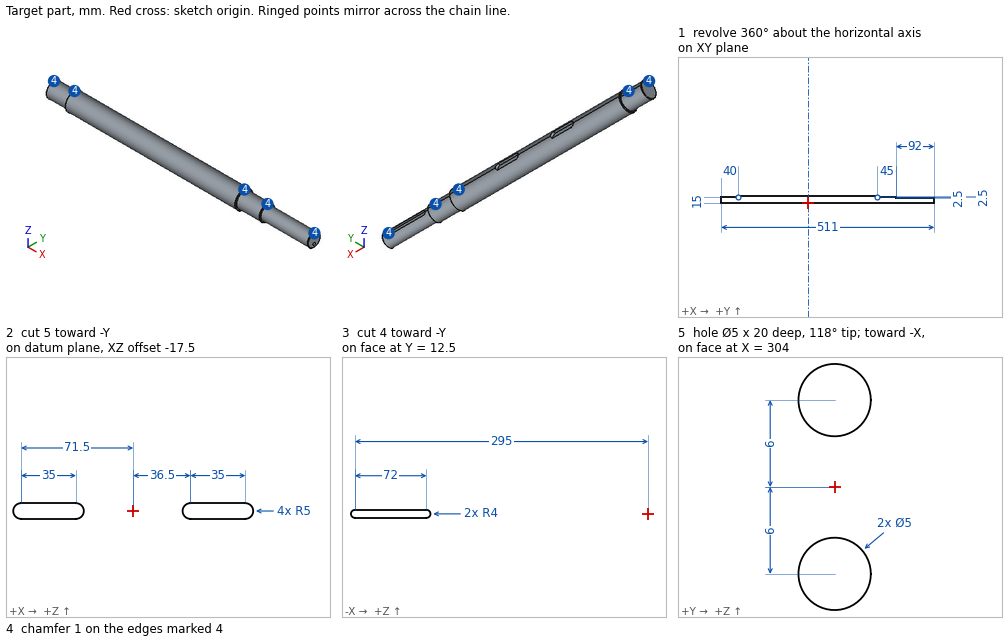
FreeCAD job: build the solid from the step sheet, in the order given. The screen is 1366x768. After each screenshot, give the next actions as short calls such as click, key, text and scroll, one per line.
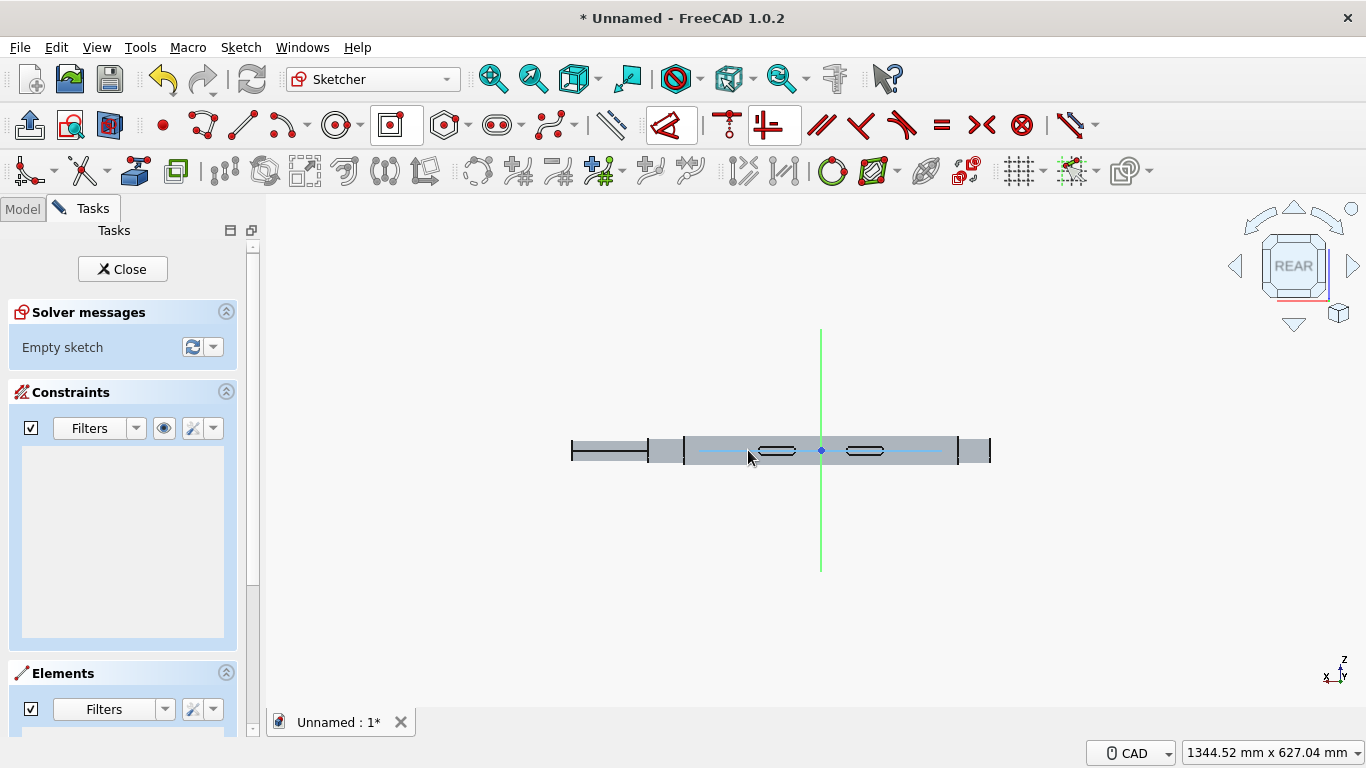
scroll(592, 451, up, 11)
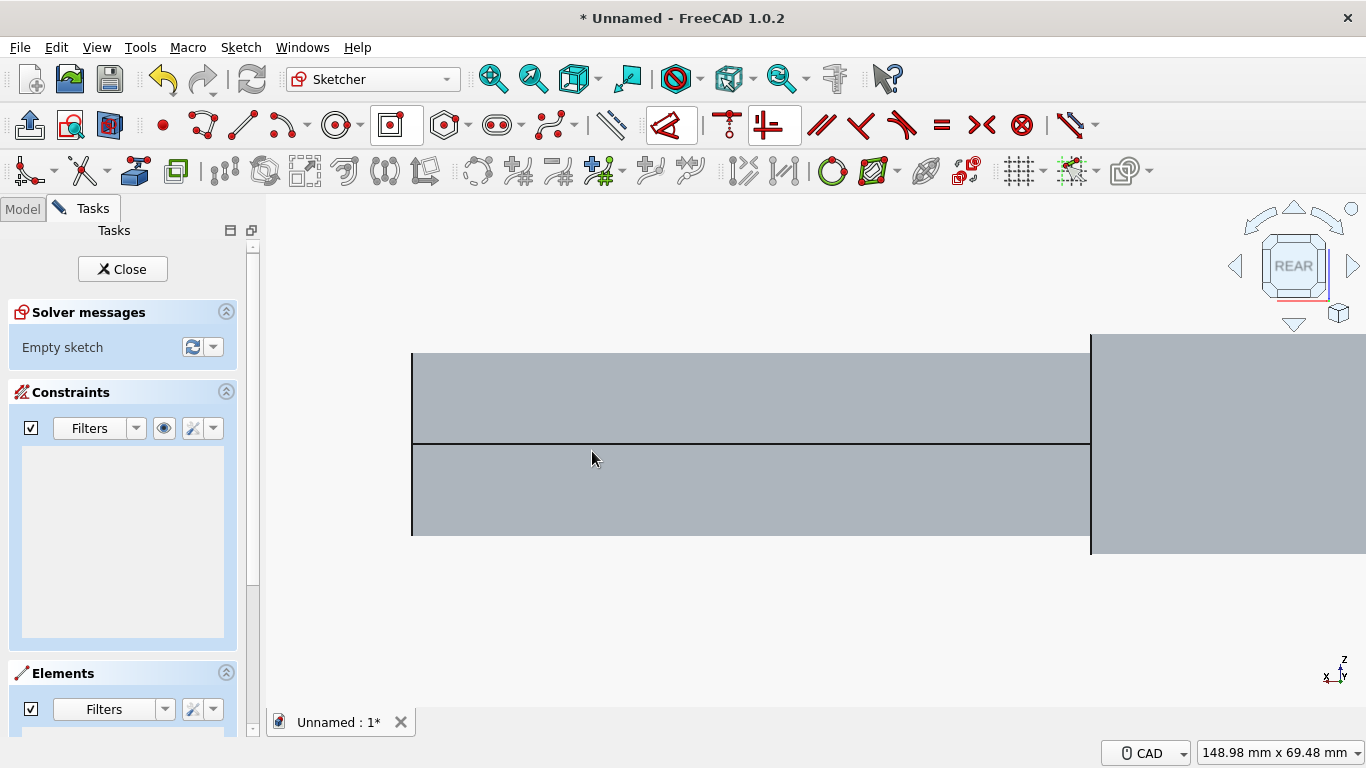
click(498, 126)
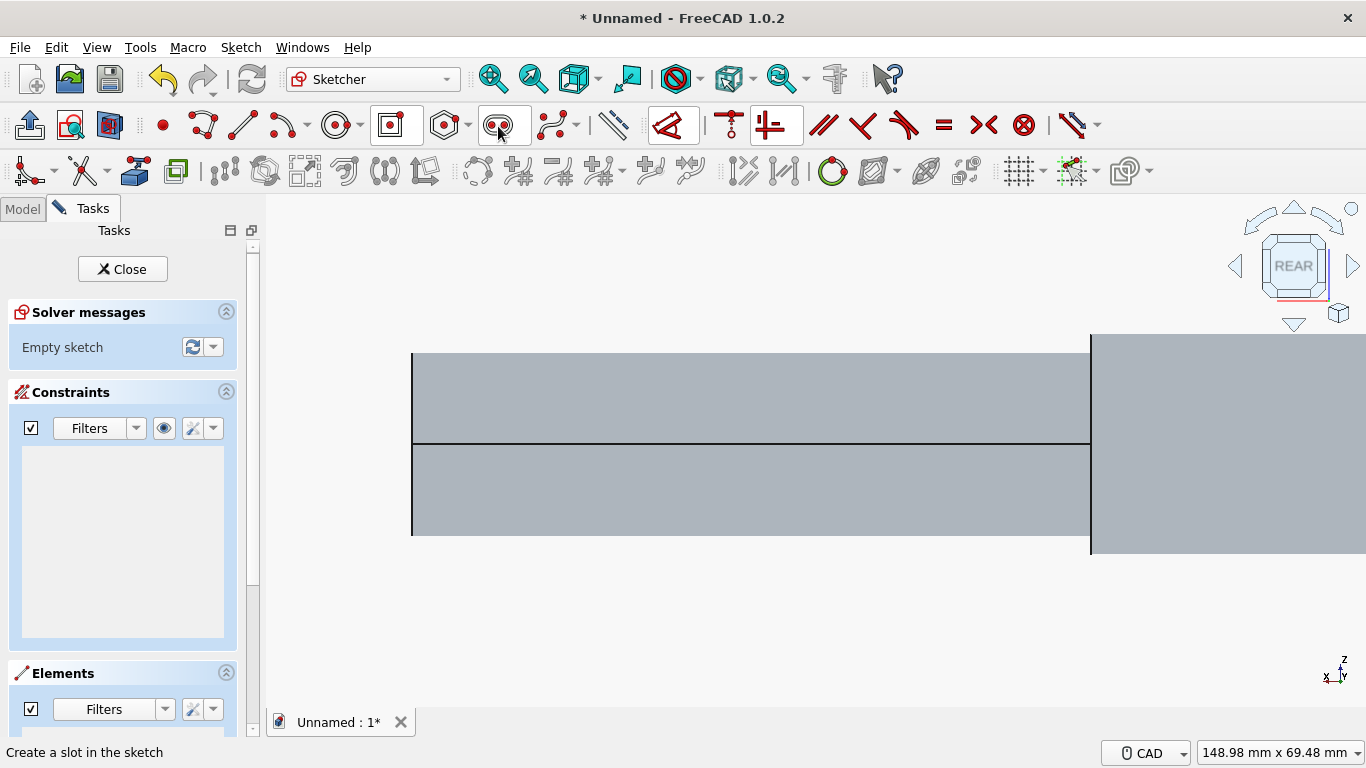
click(478, 444)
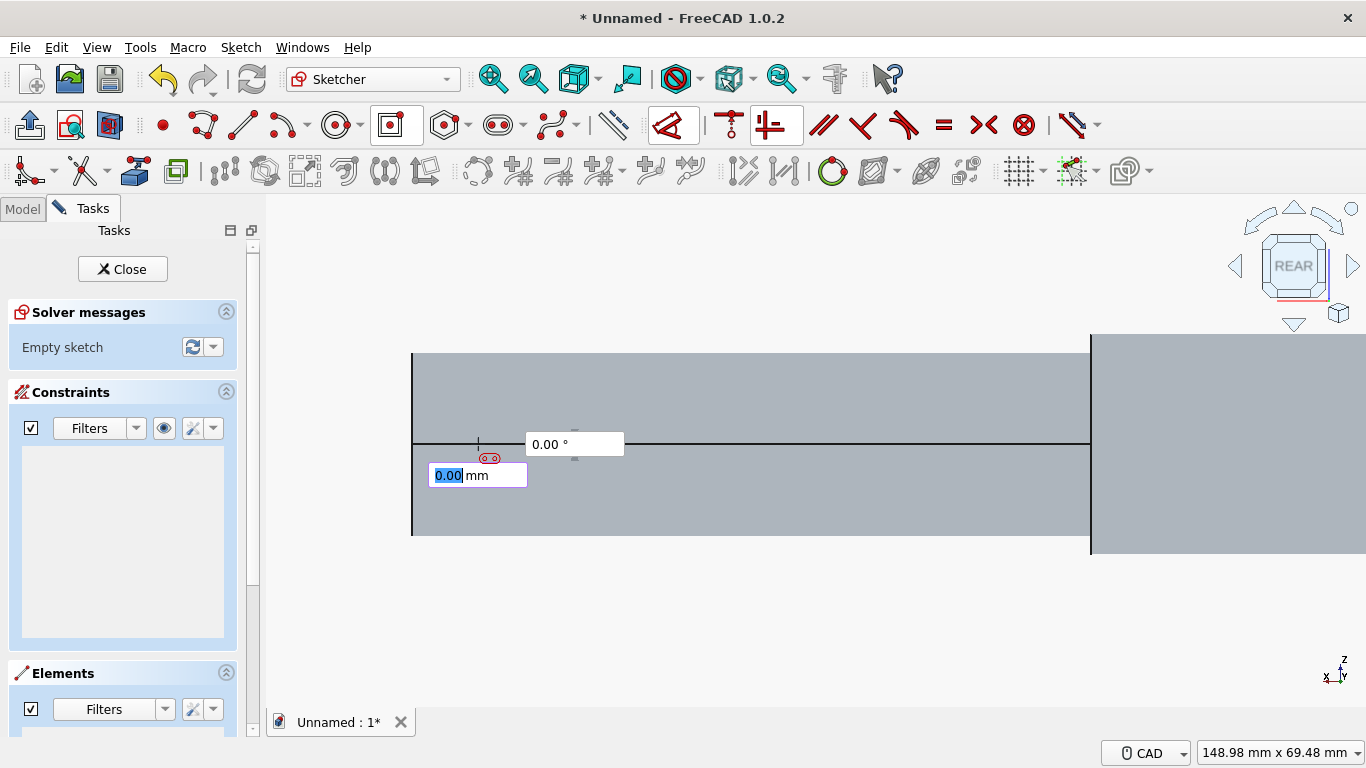
click(1010, 435)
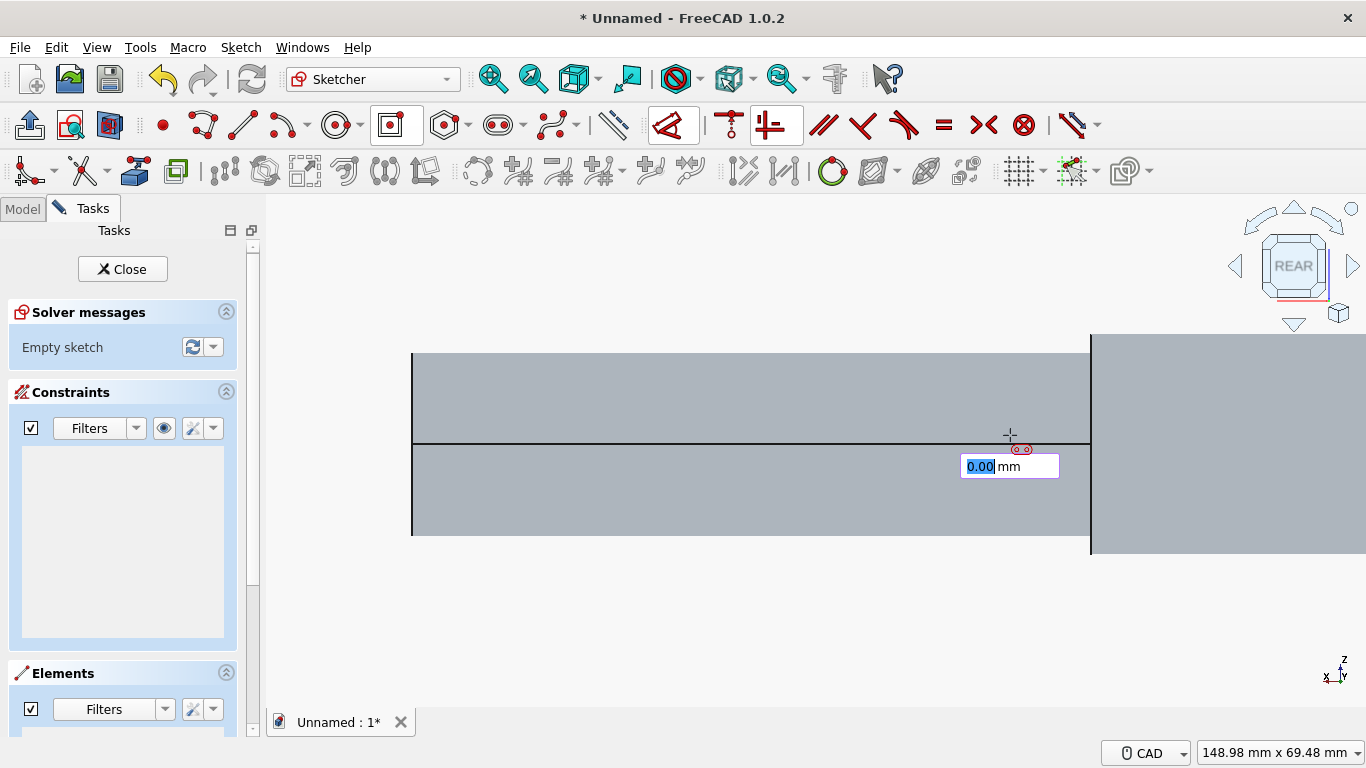
click(744, 474)
key(Escape)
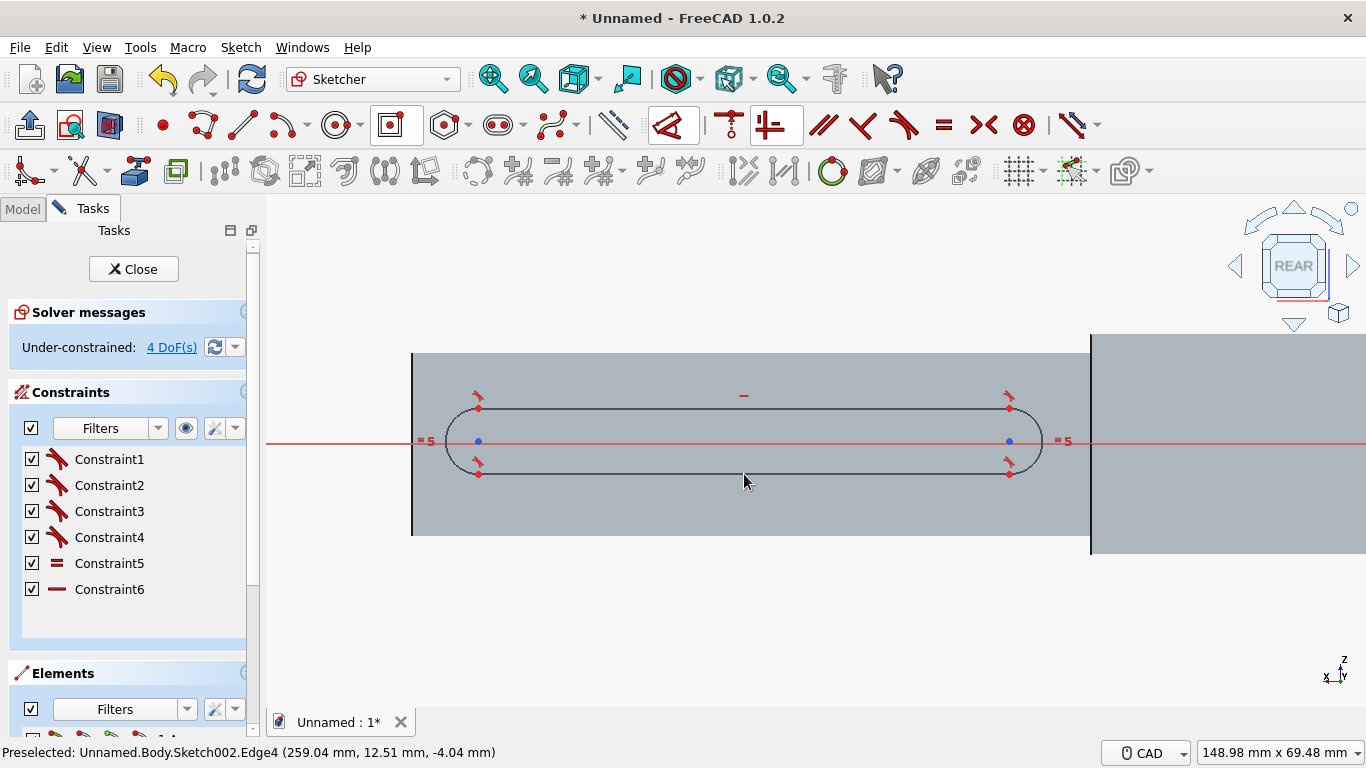
click(479, 441)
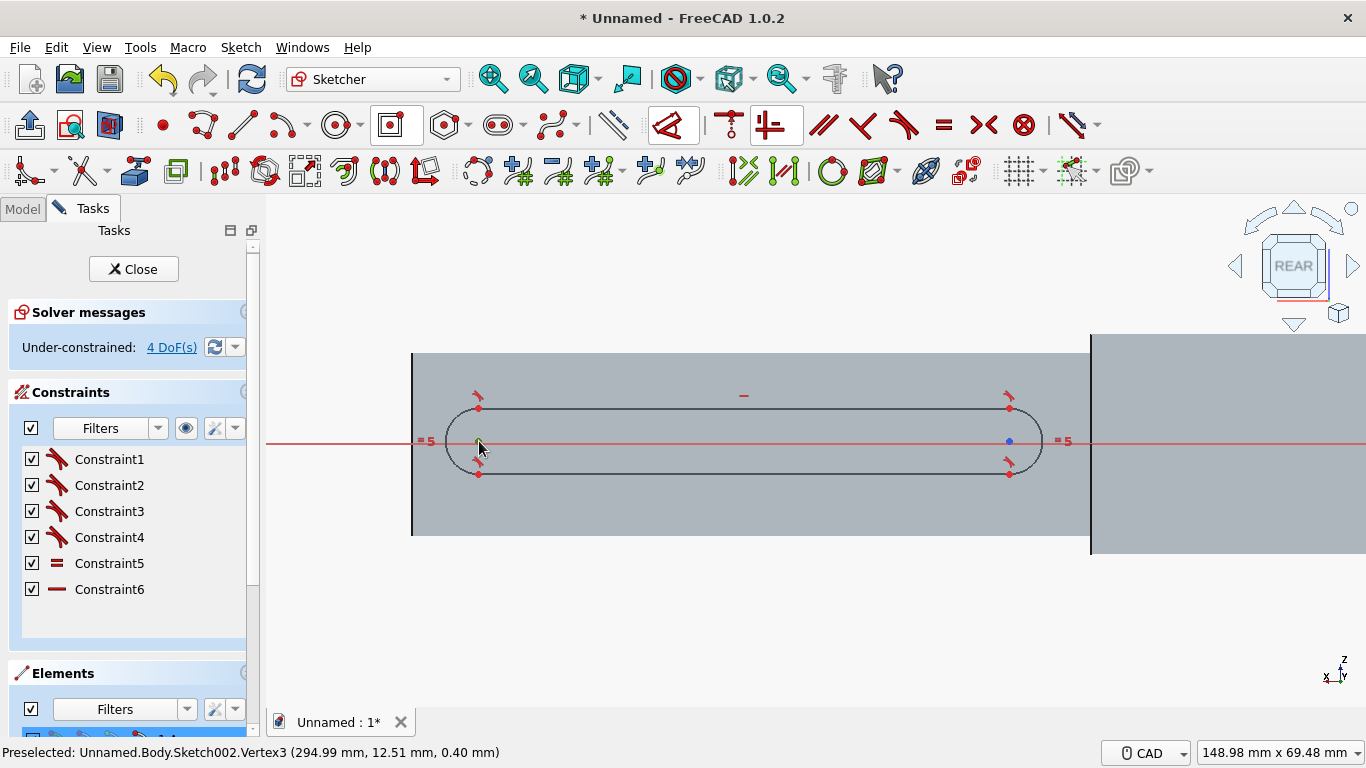
click(359, 444)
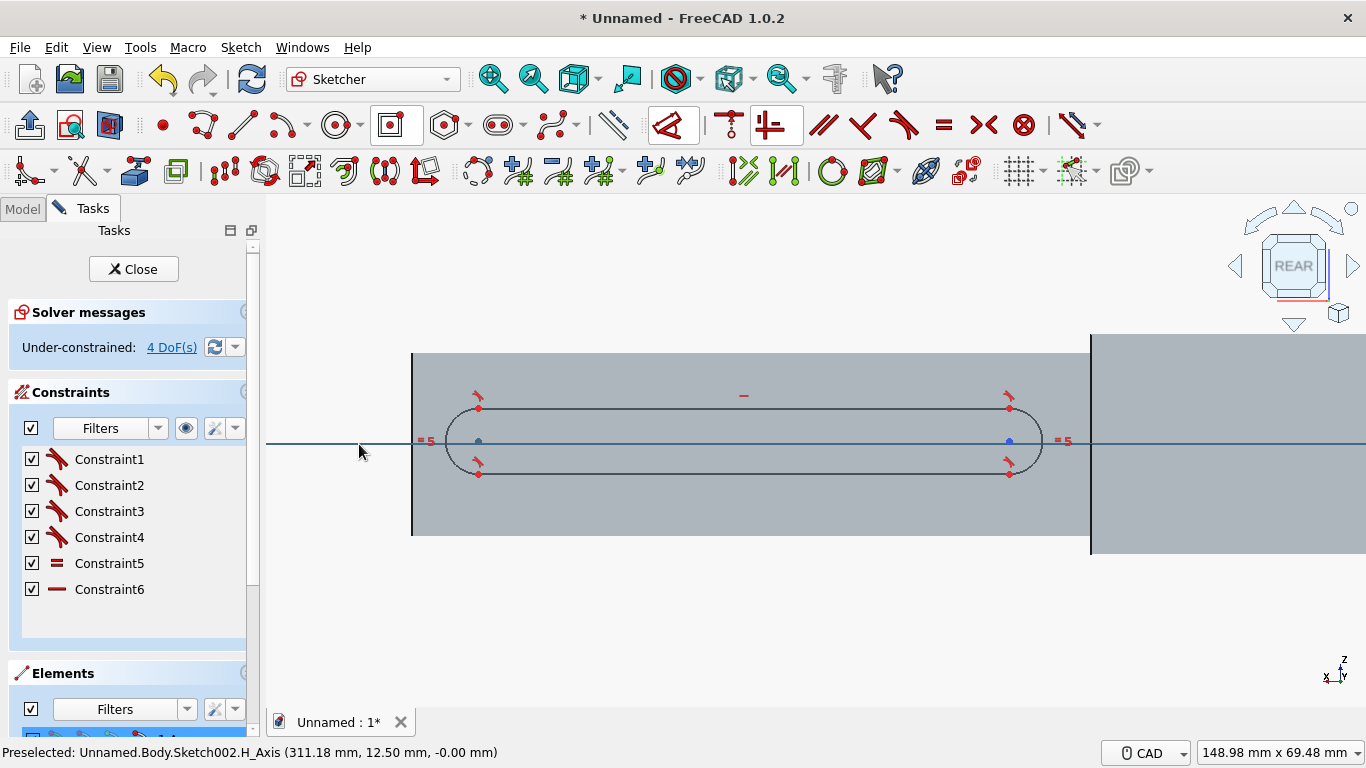
click(730, 126)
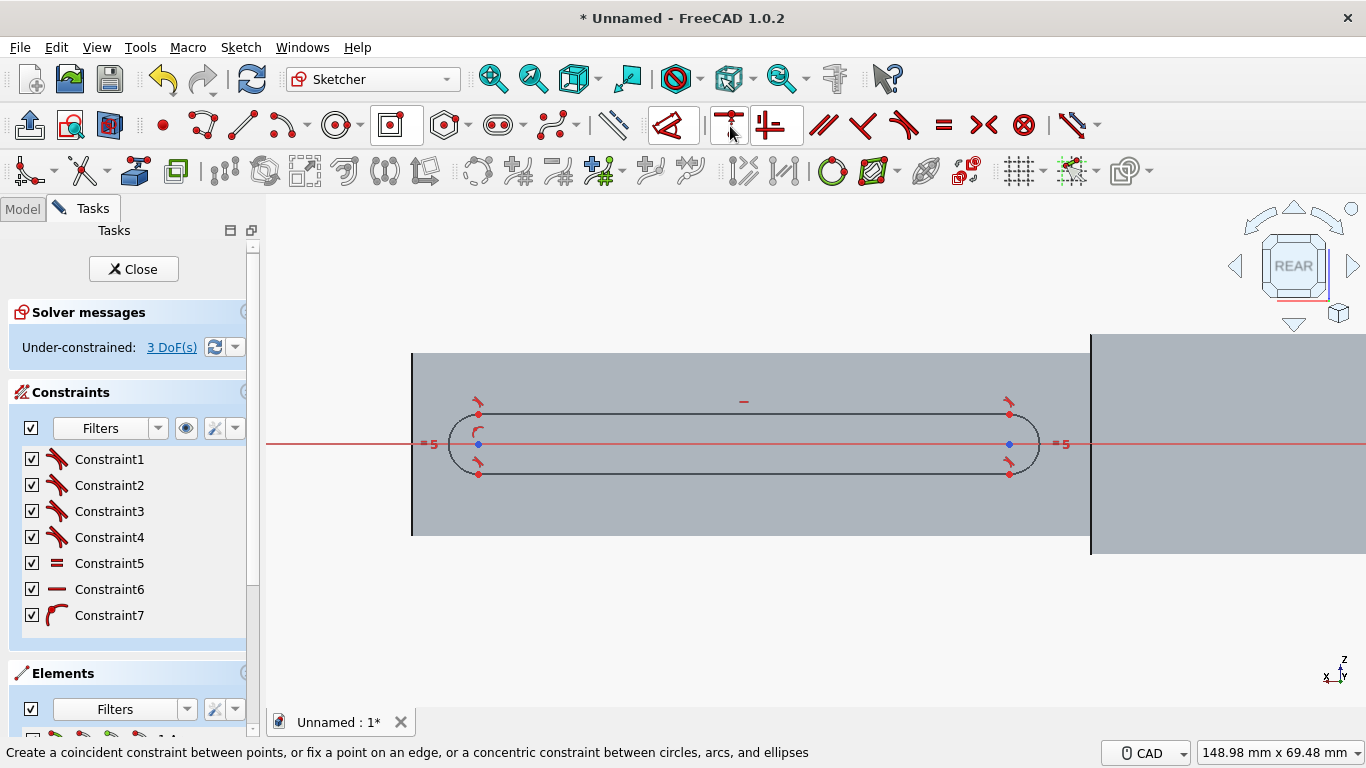
scroll(454, 427, up, 2)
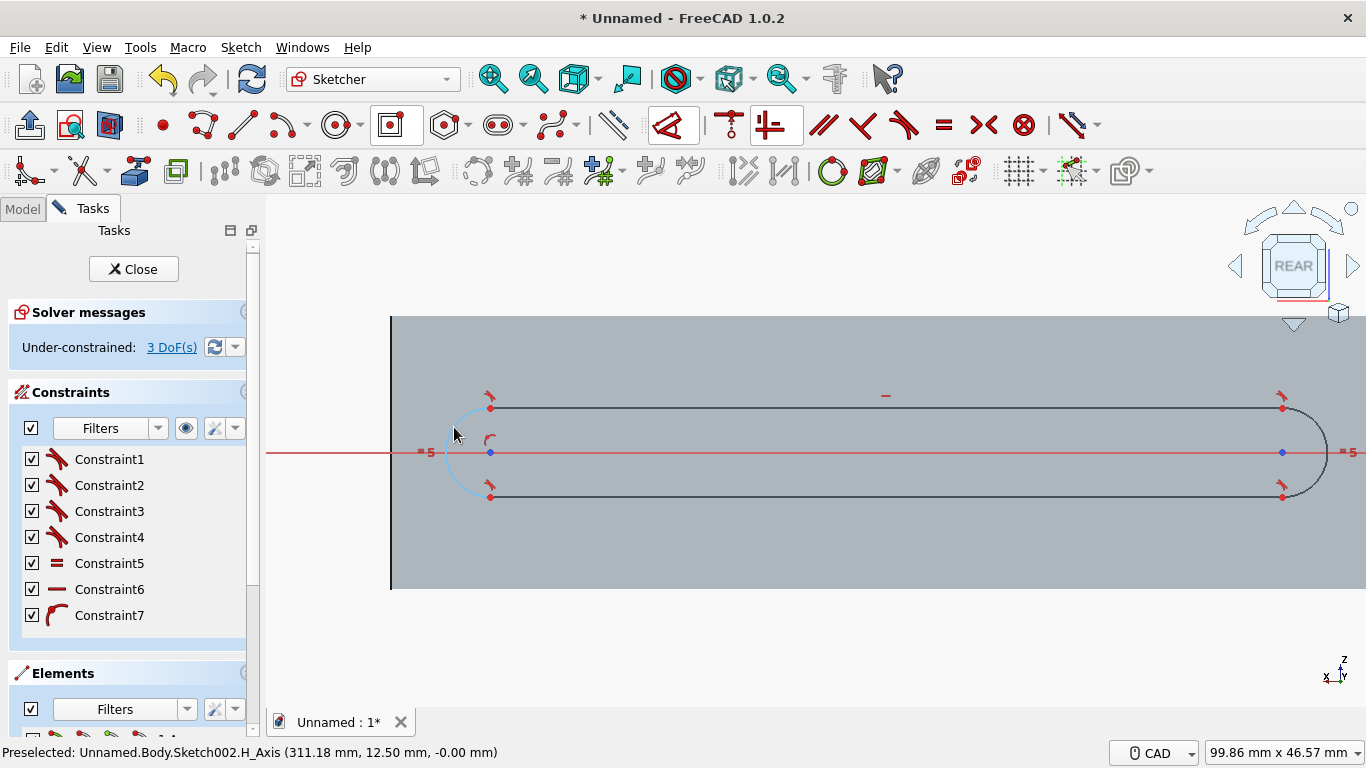
click(455, 426)